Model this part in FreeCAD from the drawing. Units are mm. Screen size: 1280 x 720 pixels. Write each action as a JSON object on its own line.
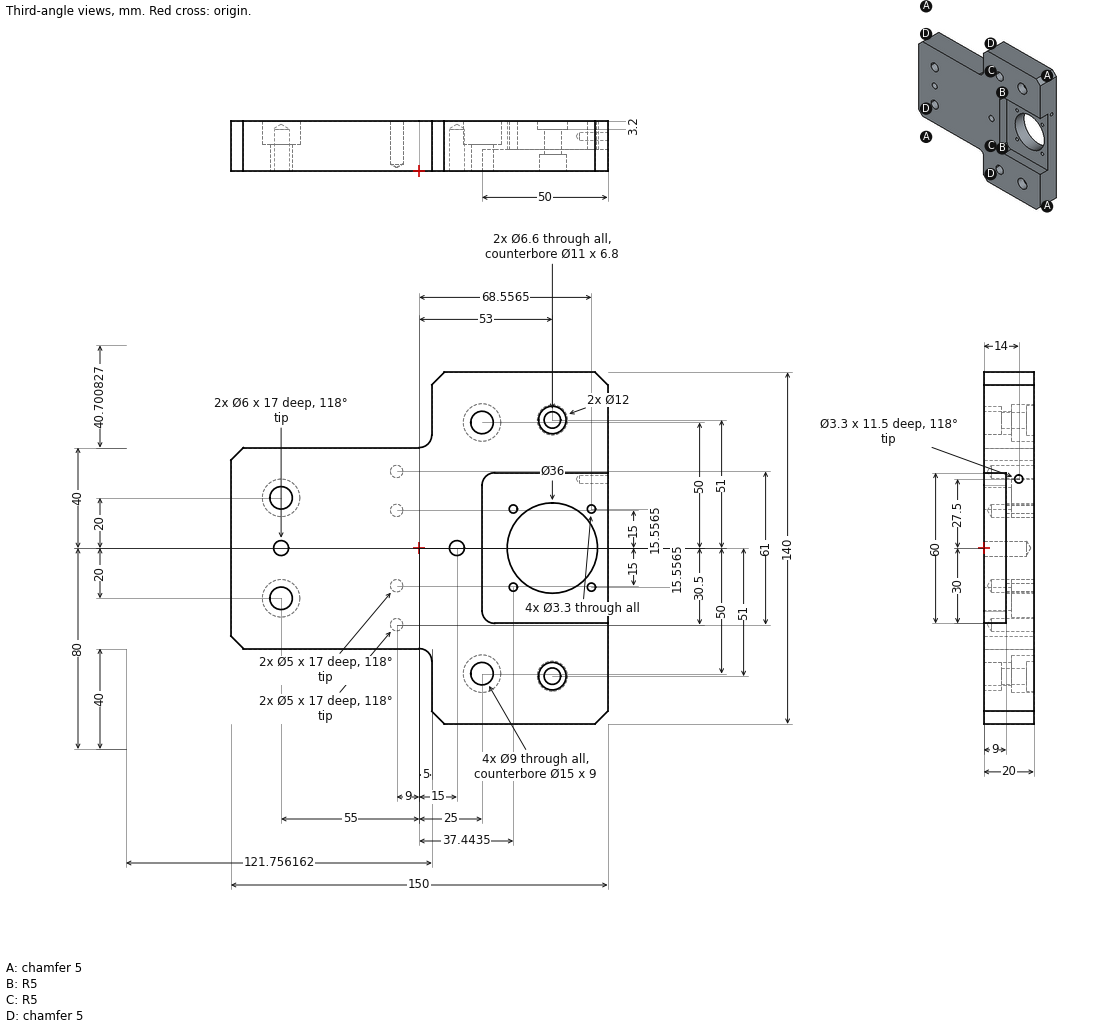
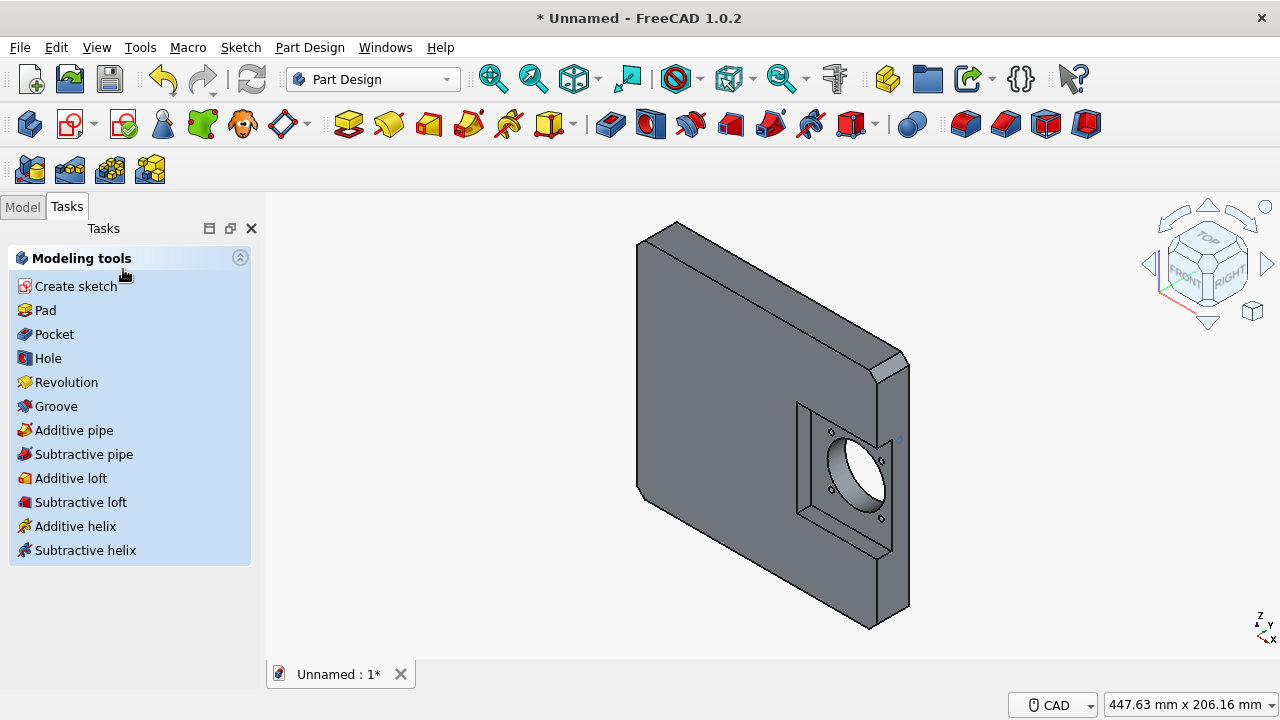
{"action": "left_click", "coordinate": [652, 124]}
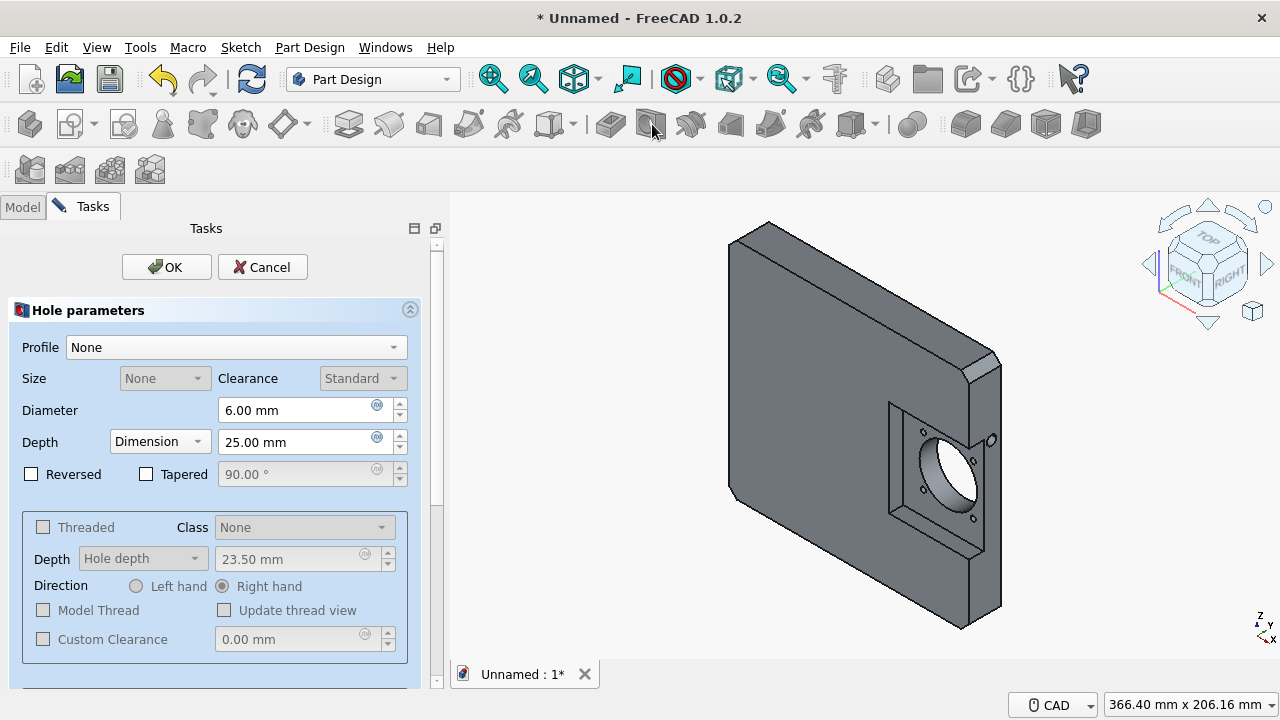
{"action": "triple_click", "coordinate": [305, 410]}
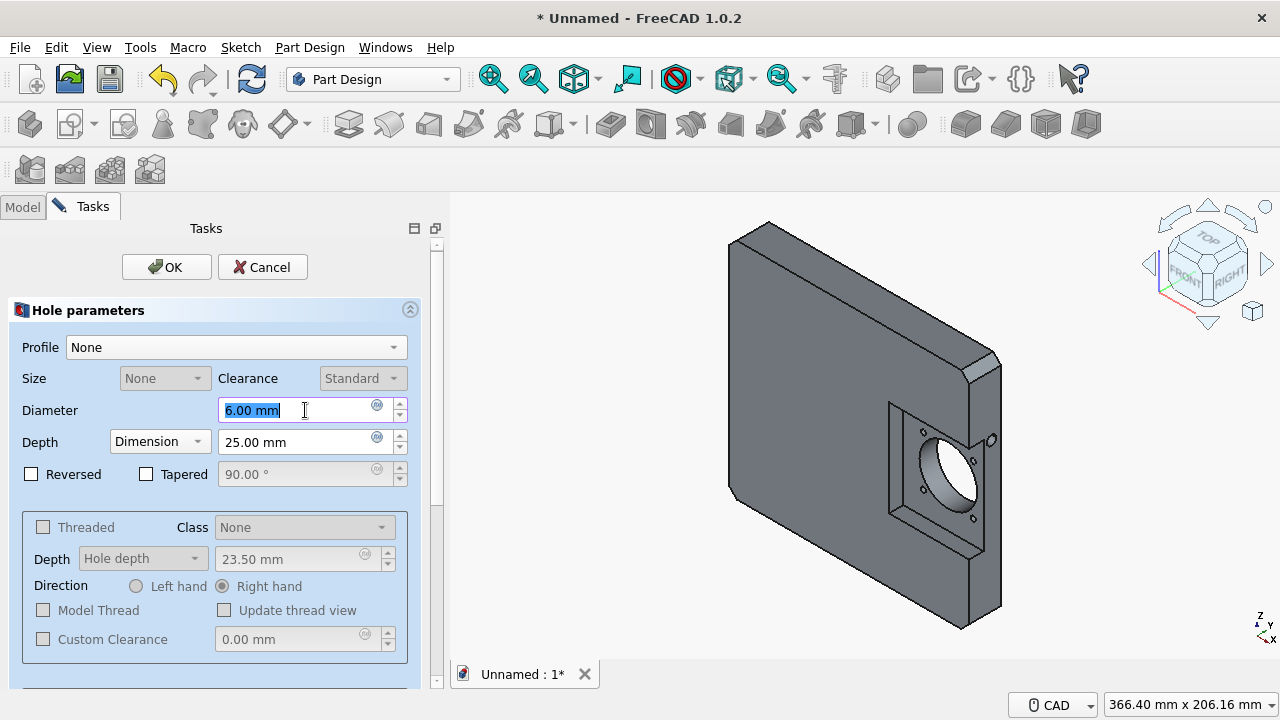
{"action": "type", "text": "3.3"}
{"action": "key", "text": "Tab"}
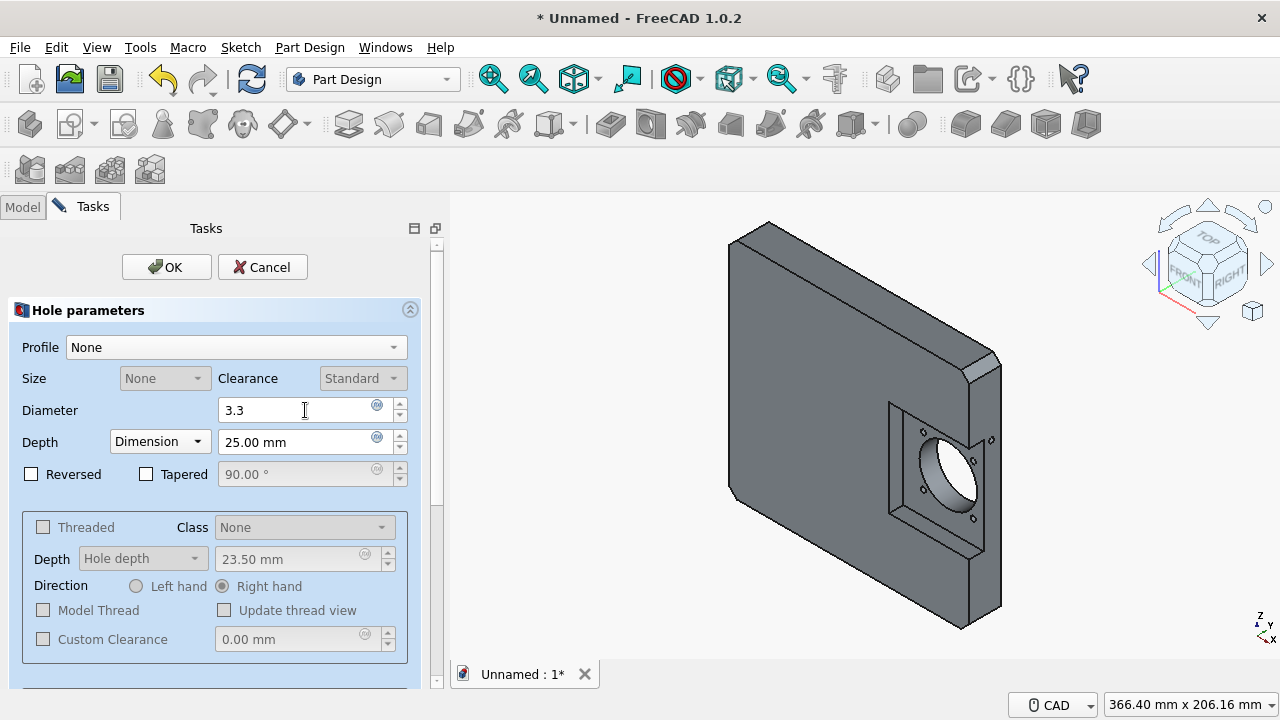
{"action": "triple_click", "coordinate": [305, 442]}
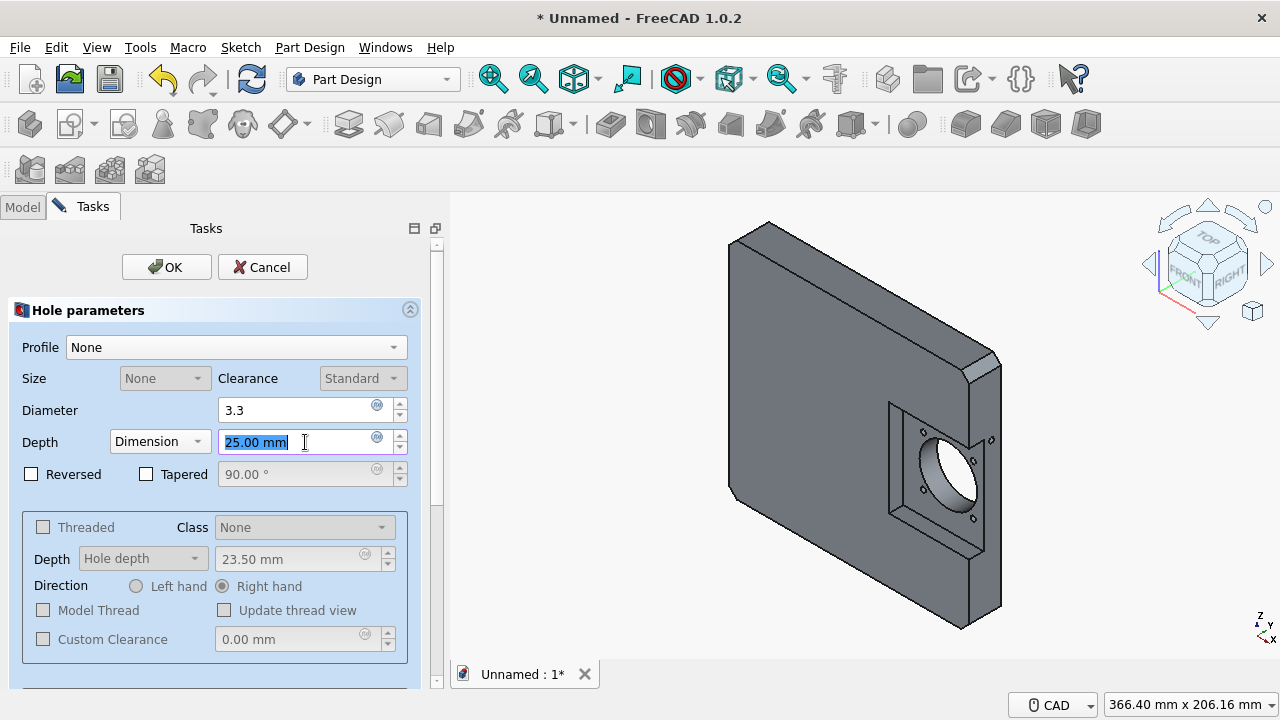
{"action": "type", "text": "11.5"}
{"action": "key", "text": "Tab"}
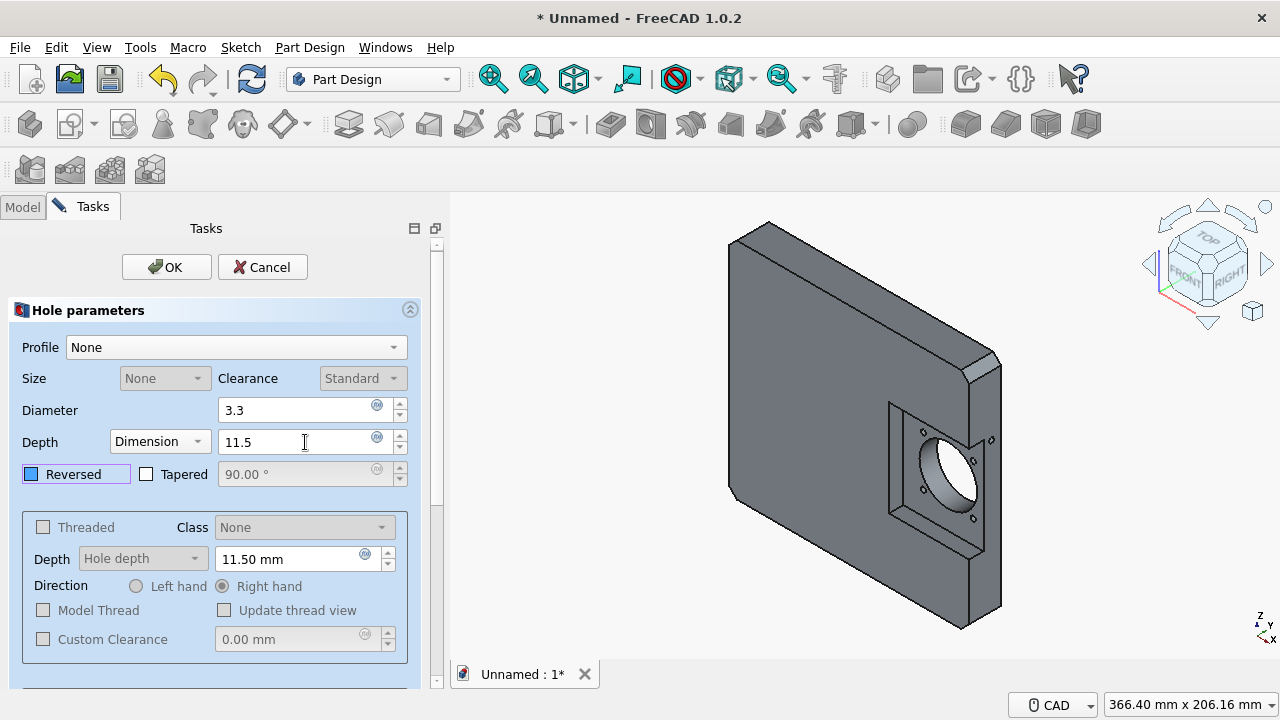
{"action": "left_click", "coordinate": [167, 267]}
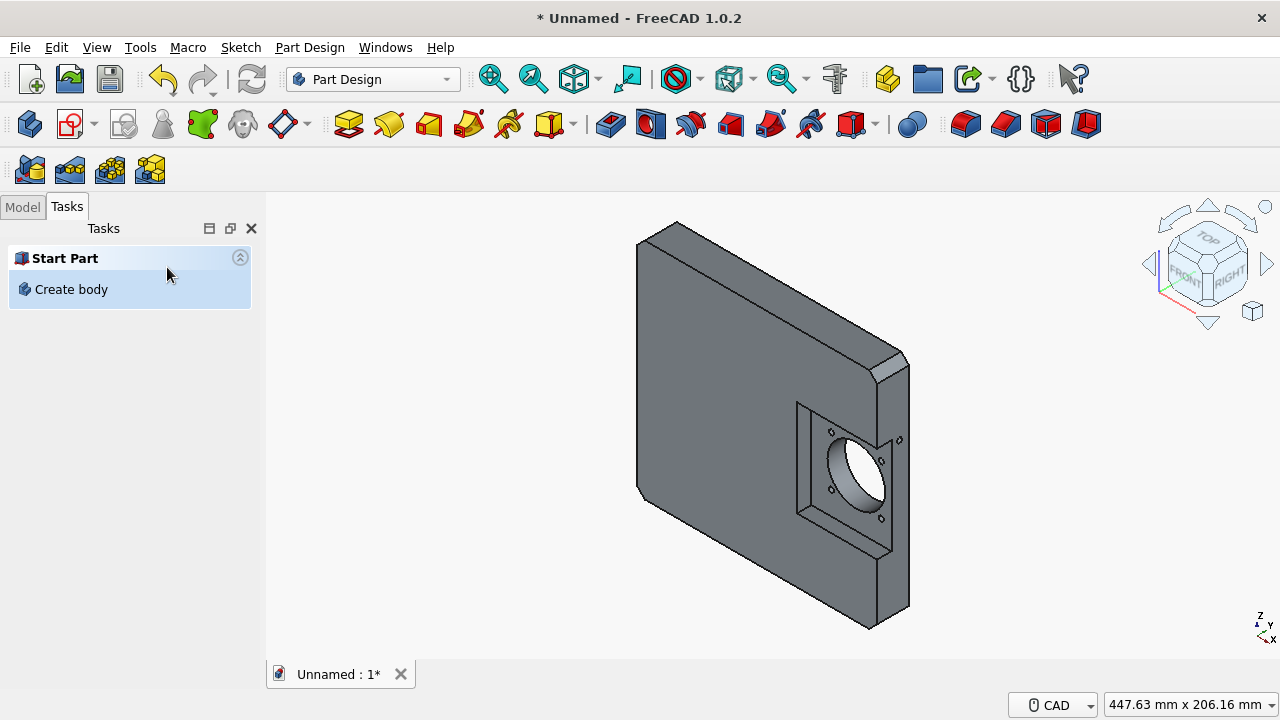
{"action": "scroll", "coordinate": [804, 397], "scroll_direction": "up", "scroll_amount": 4}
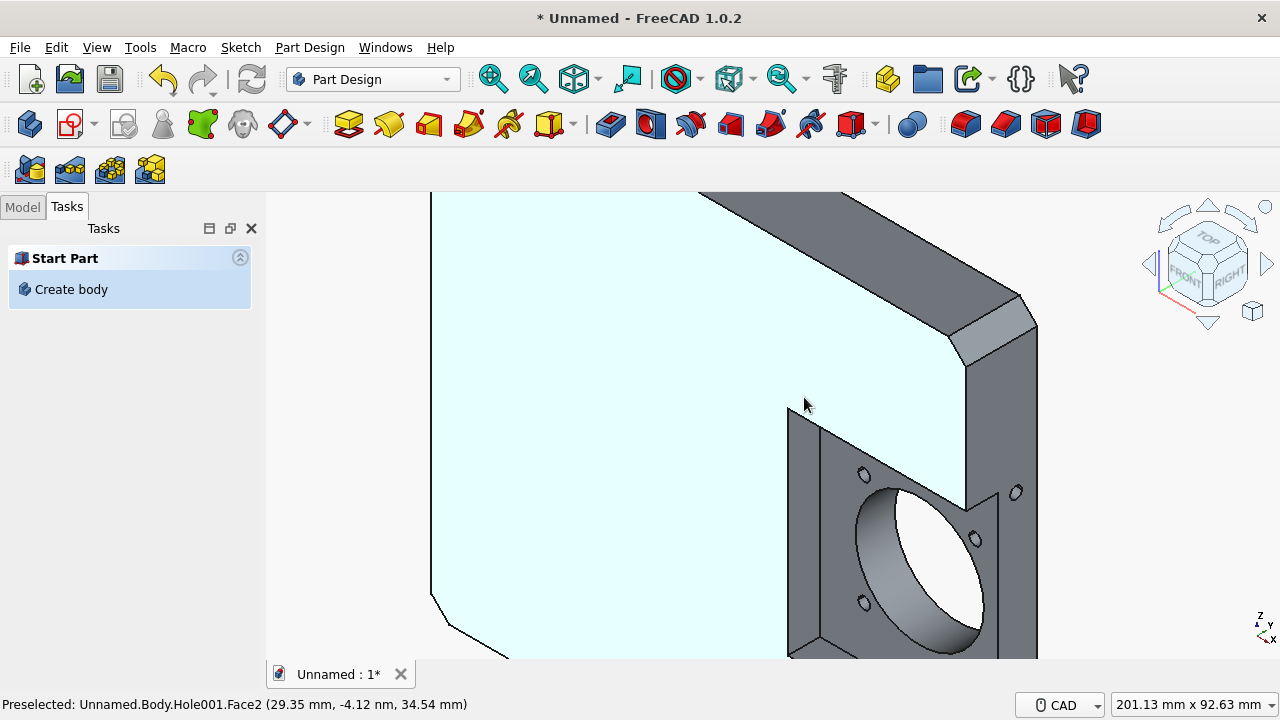
{"action": "left_click", "coordinate": [494, 80]}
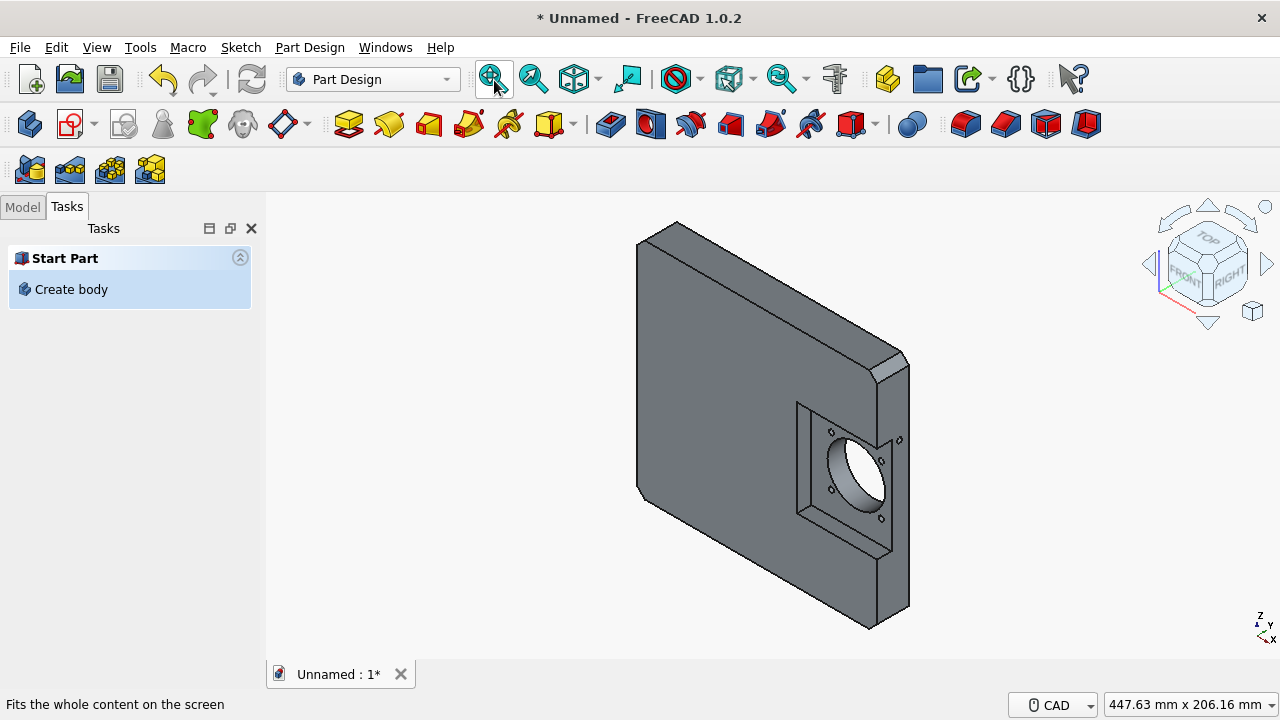
{"action": "key", "text": "2"}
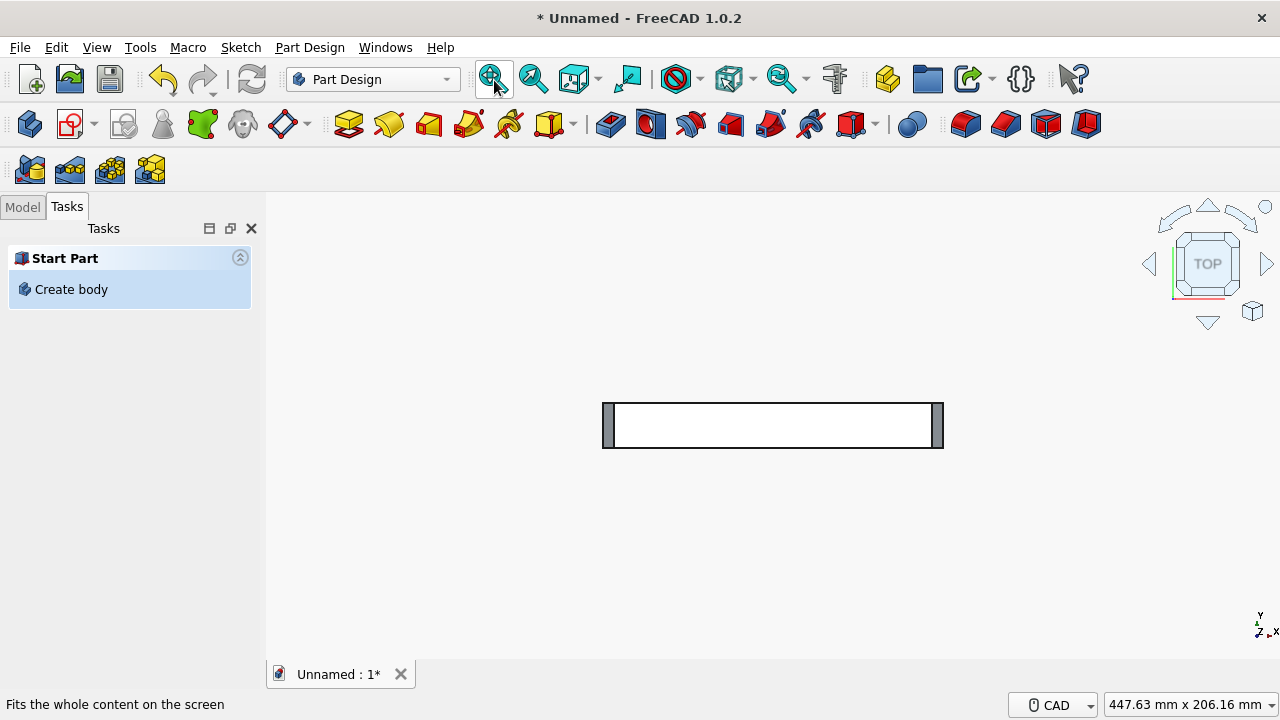
{"action": "left_click", "coordinate": [494, 80]}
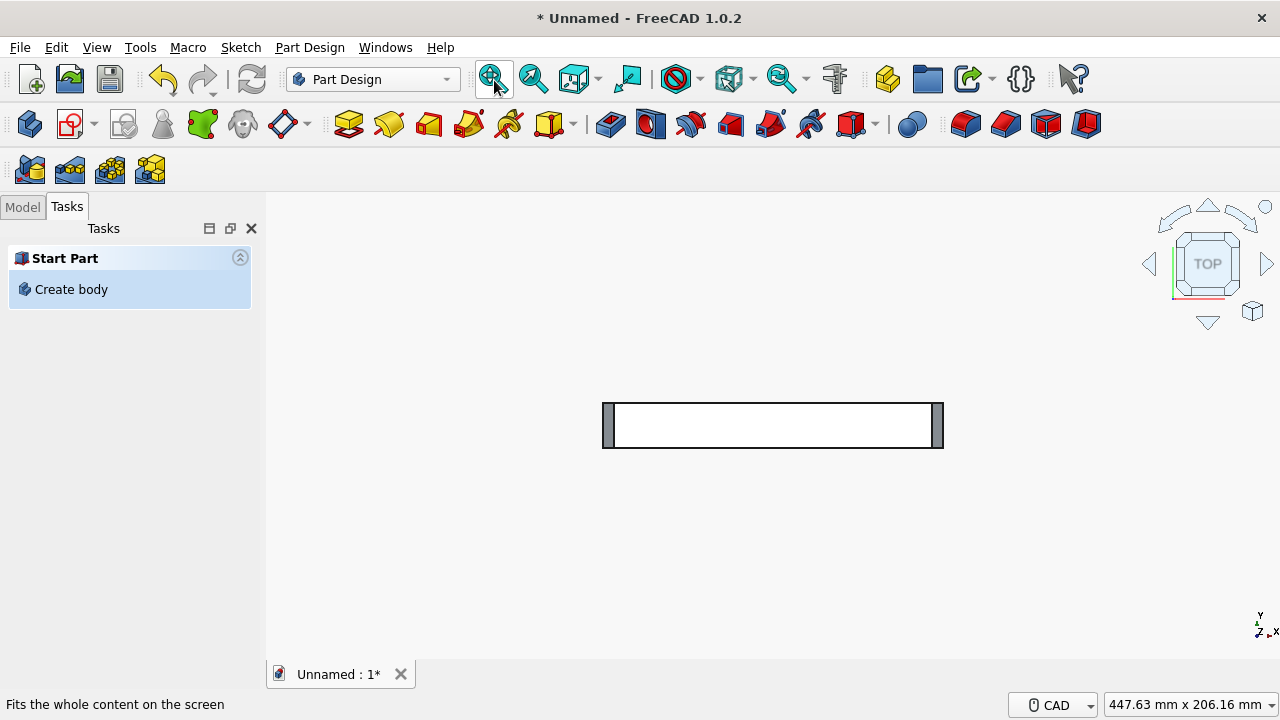
{"action": "scroll", "coordinate": [830, 437], "scroll_direction": "up", "scroll_amount": 4}